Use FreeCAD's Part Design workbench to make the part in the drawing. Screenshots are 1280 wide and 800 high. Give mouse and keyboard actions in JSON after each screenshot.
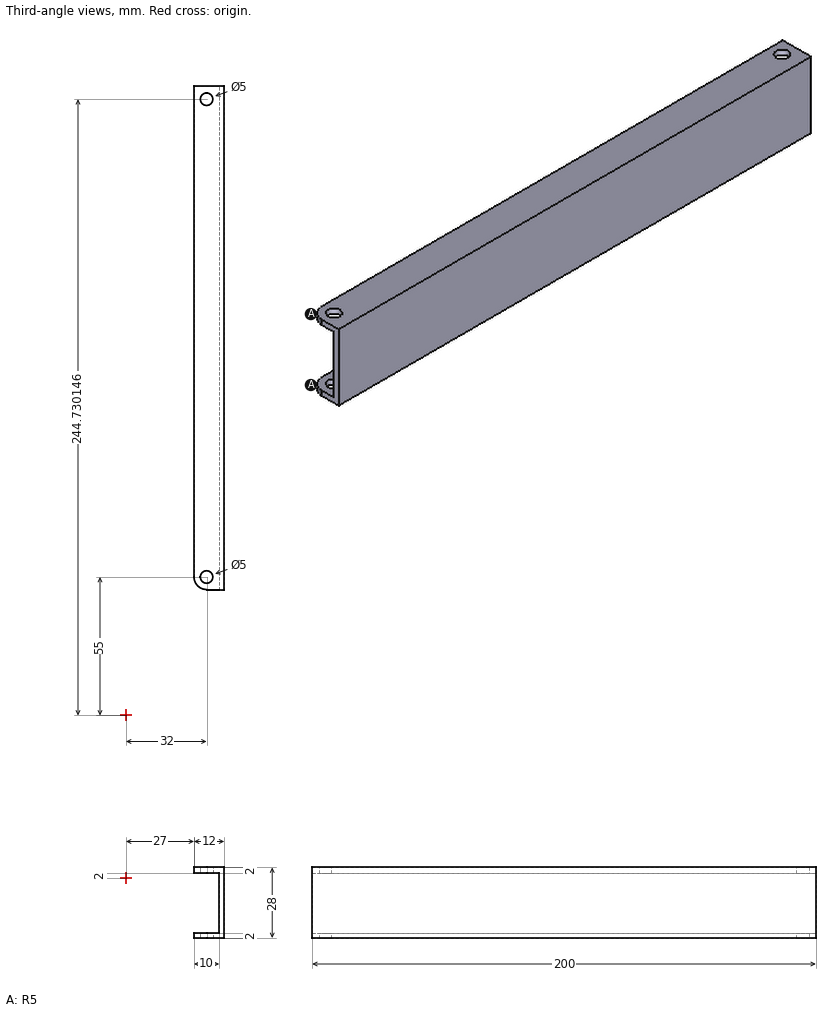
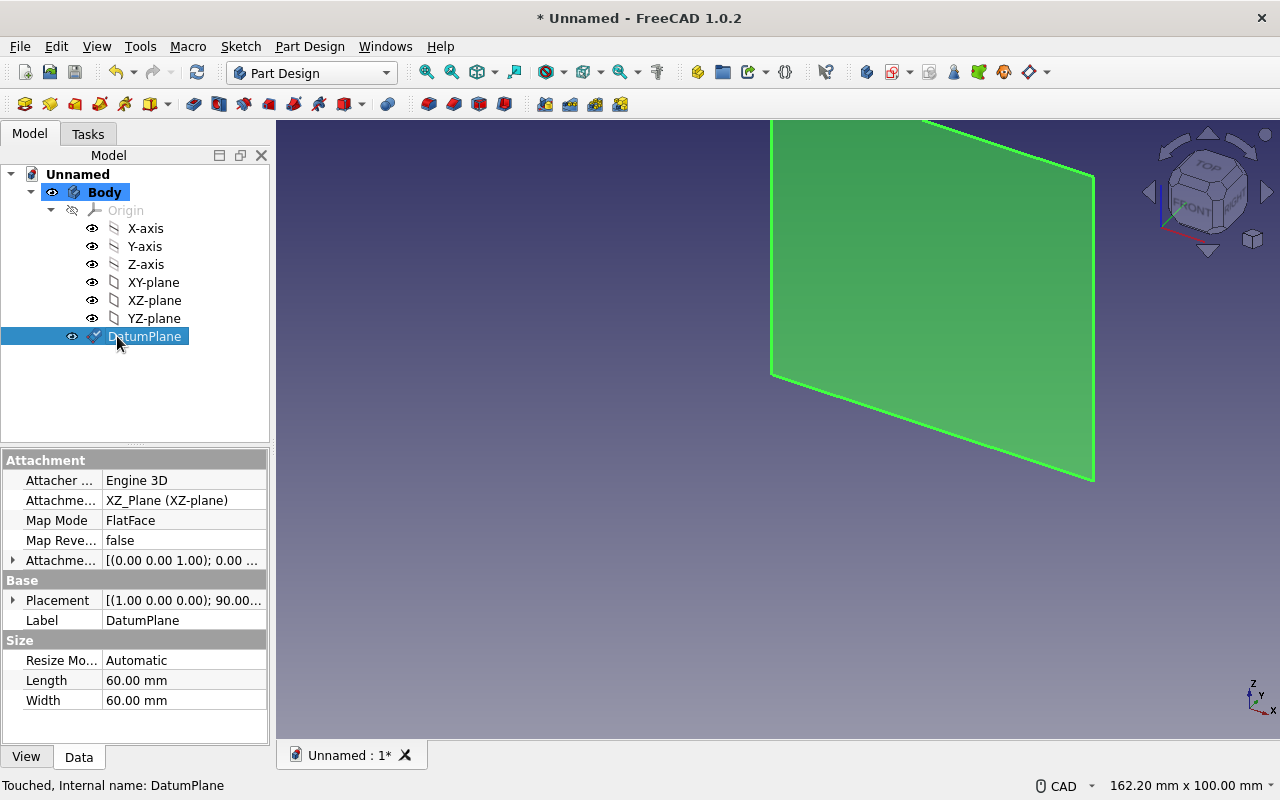
{"action": "left_click", "coordinate": [892, 72]}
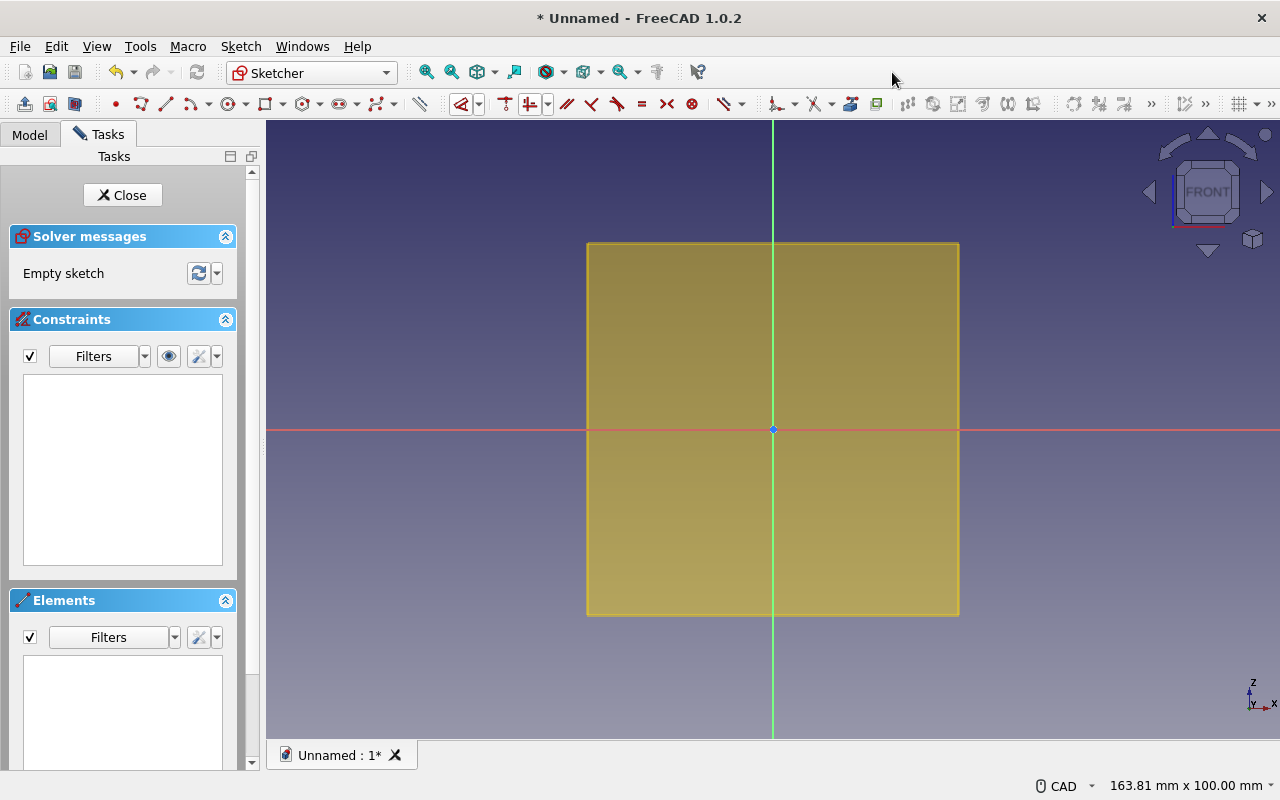
{"action": "scroll", "coordinate": [1048, 542], "scroll_direction": "up", "scroll_amount": 4}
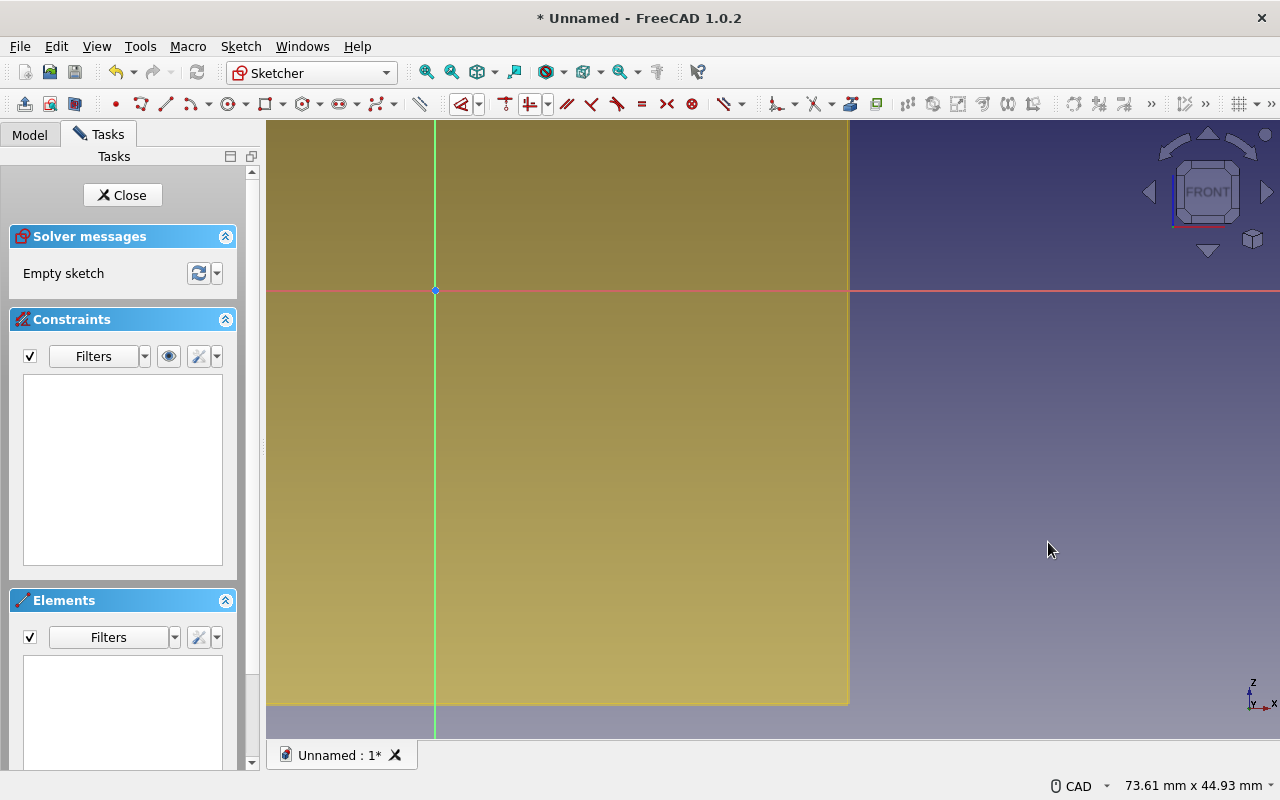
{"action": "left_click", "coordinate": [141, 104]}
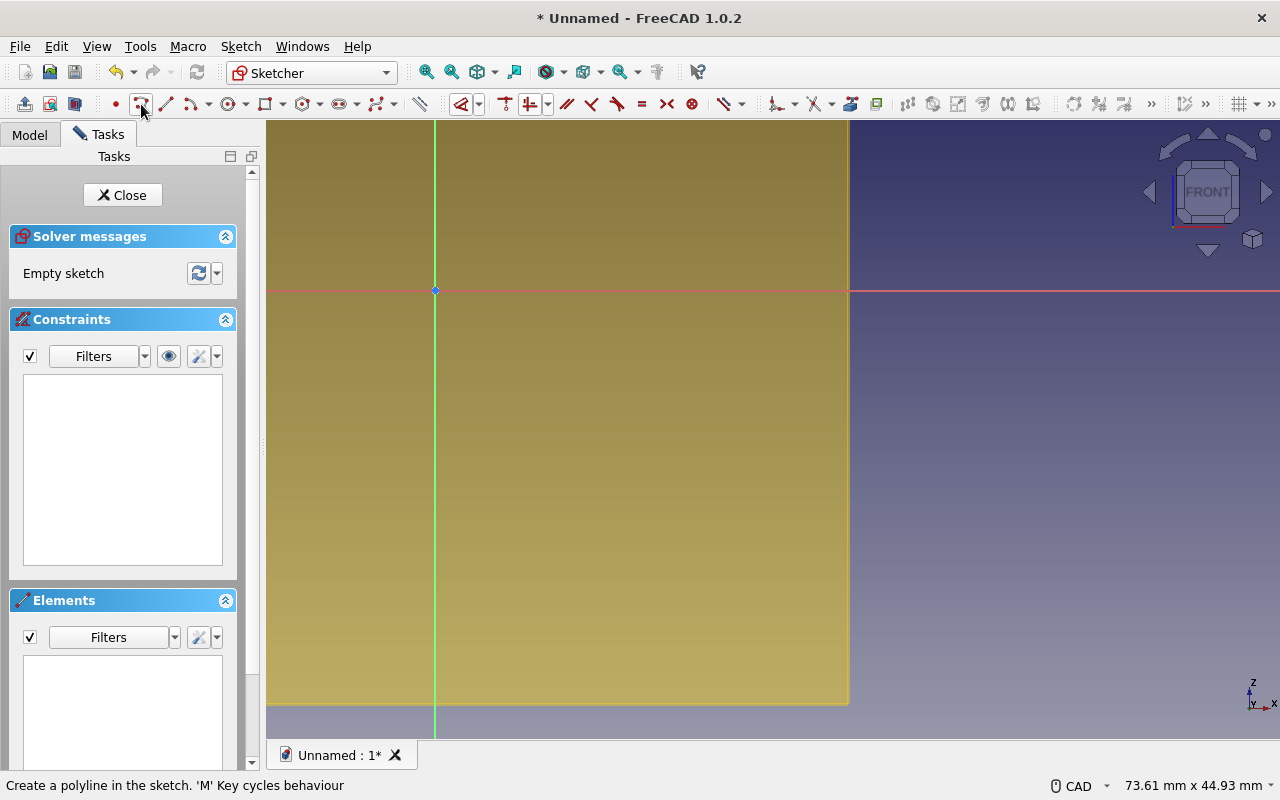
{"action": "left_click", "coordinate": [807, 263]}
{"action": "left_click", "coordinate": [807, 236]}
{"action": "left_click", "coordinate": [972, 236]}
{"action": "left_click", "coordinate": [972, 621]}
{"action": "left_click", "coordinate": [807, 621]}
{"action": "left_click", "coordinate": [807, 594]}
{"action": "left_click", "coordinate": [945, 594]}
{"action": "left_click", "coordinate": [945, 263]}
{"action": "left_click", "coordinate": [807, 264]}
{"action": "key", "text": "Escape"}
{"action": "key", "text": "Escape"}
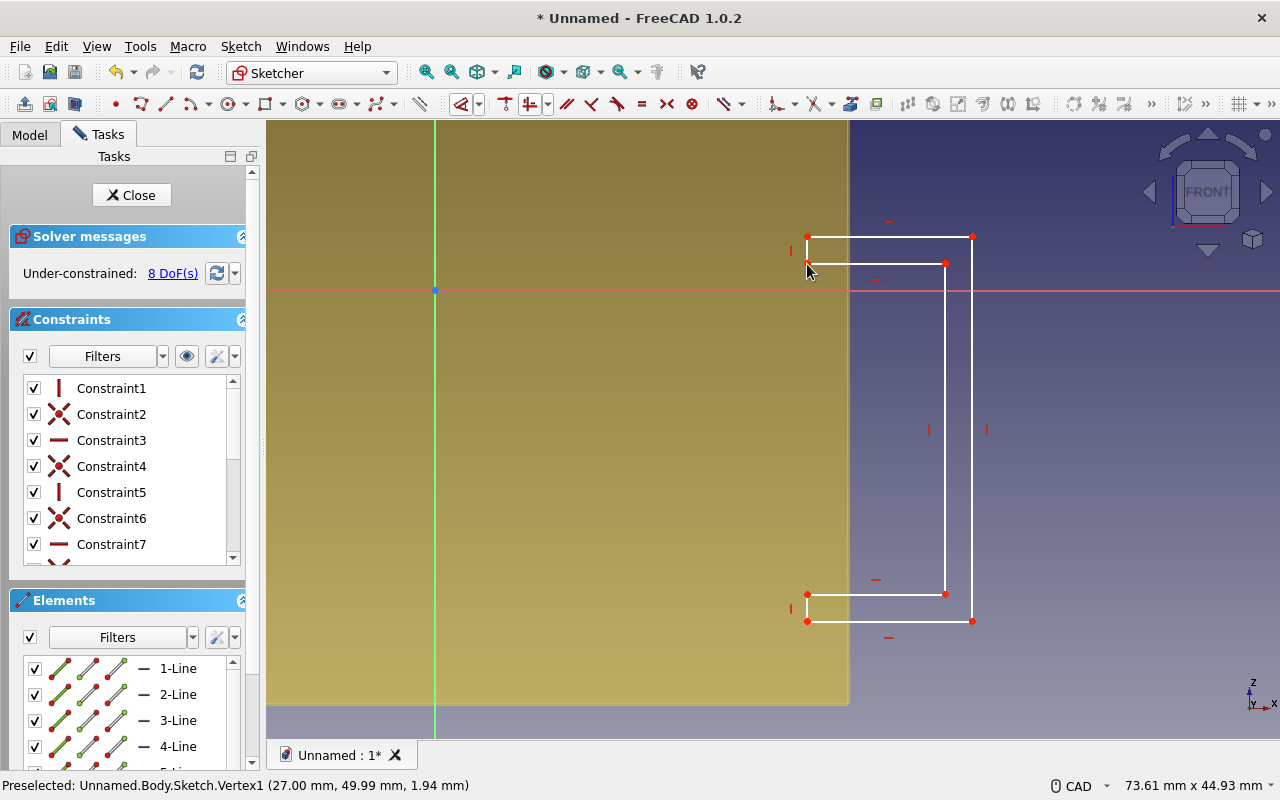
{"action": "scroll", "coordinate": [807, 253], "scroll_direction": "up", "scroll_amount": 2}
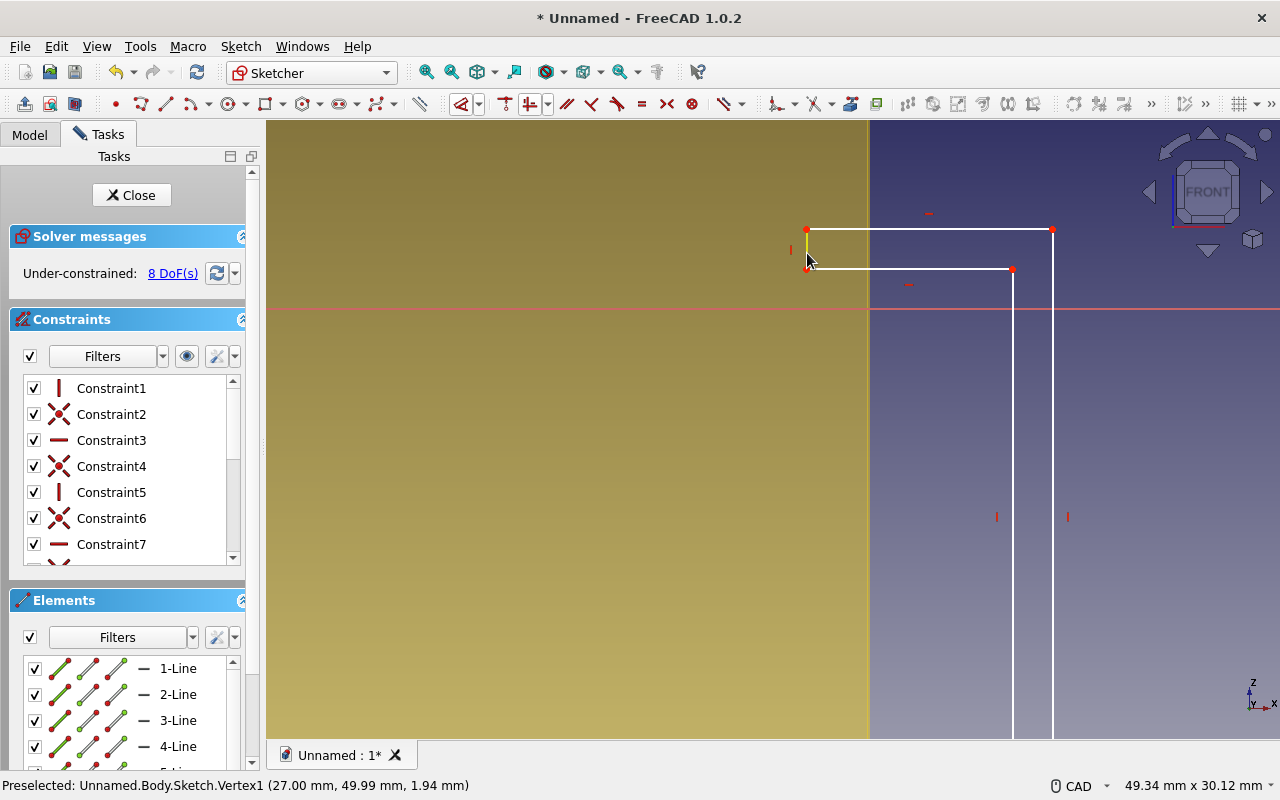
{"action": "left_click", "coordinate": [807, 253]}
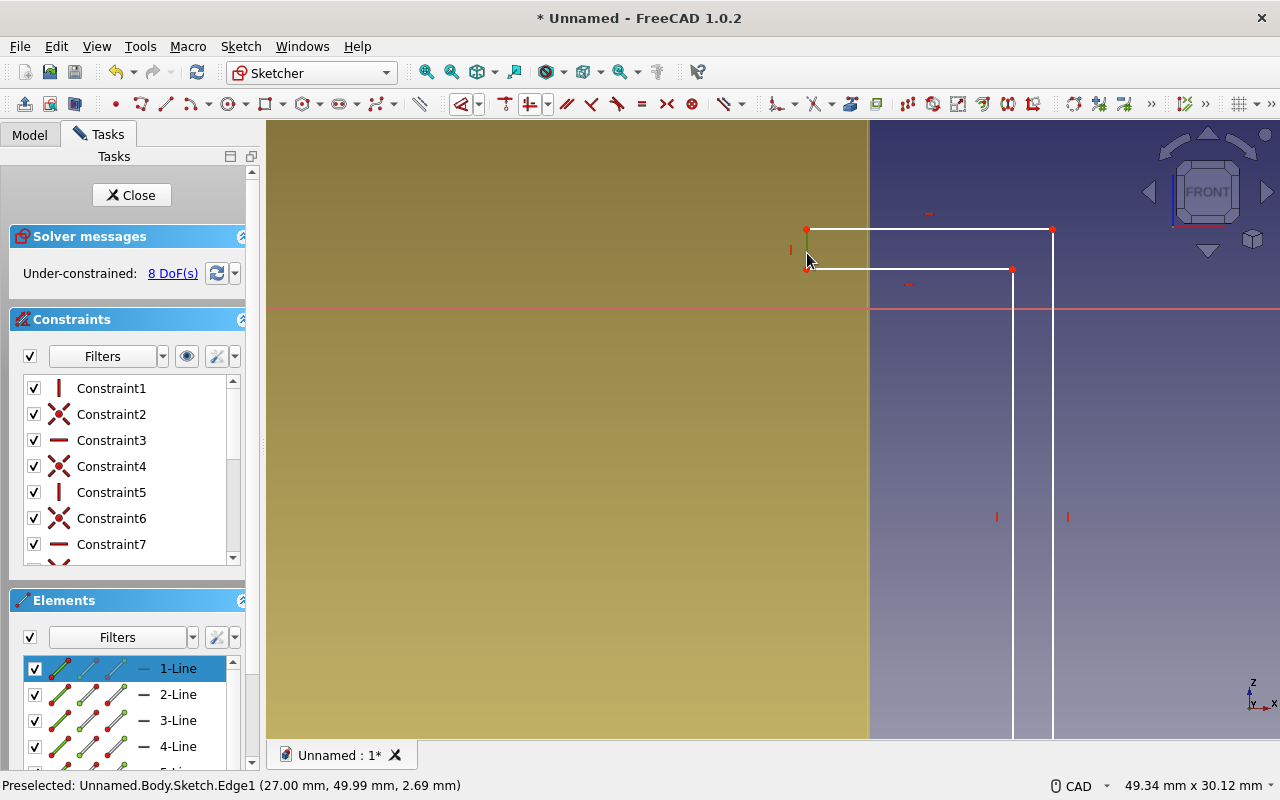
{"action": "left_click", "coordinate": [478, 104]}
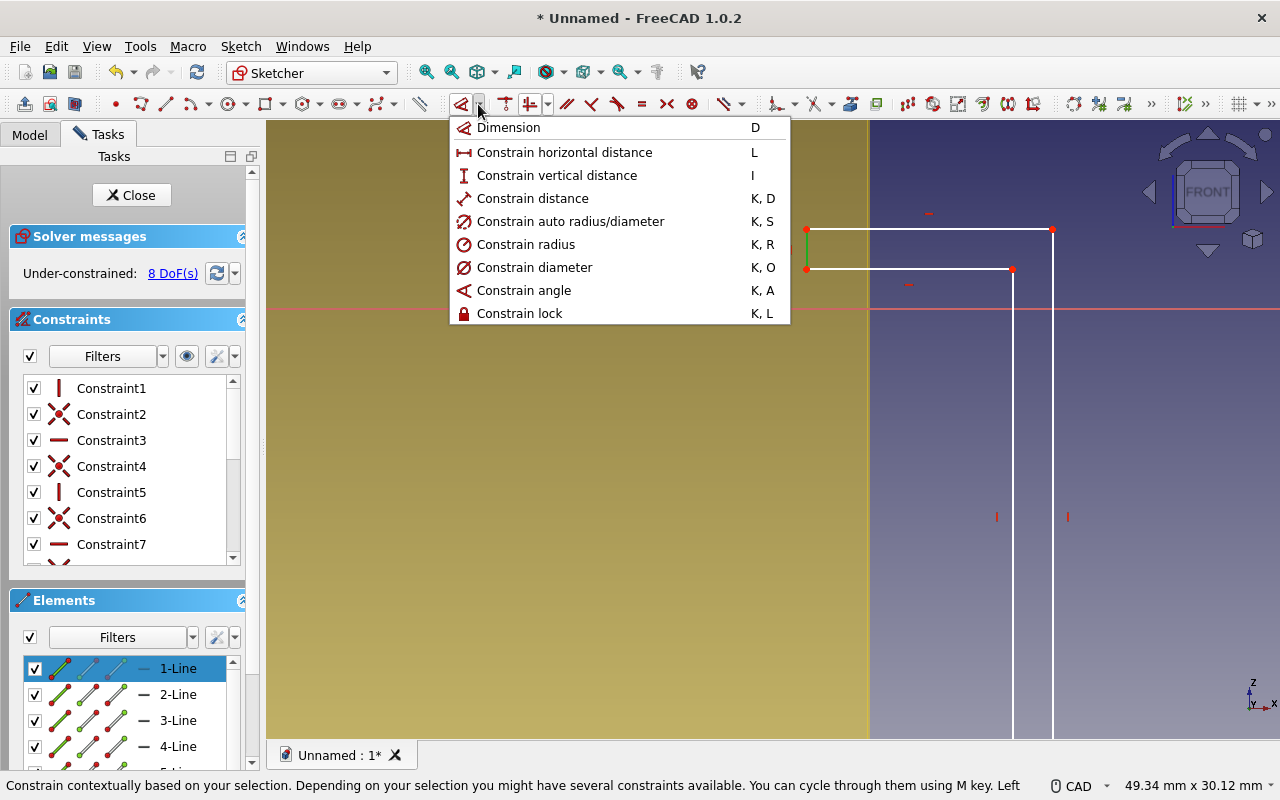
{"action": "left_click", "coordinate": [620, 176]}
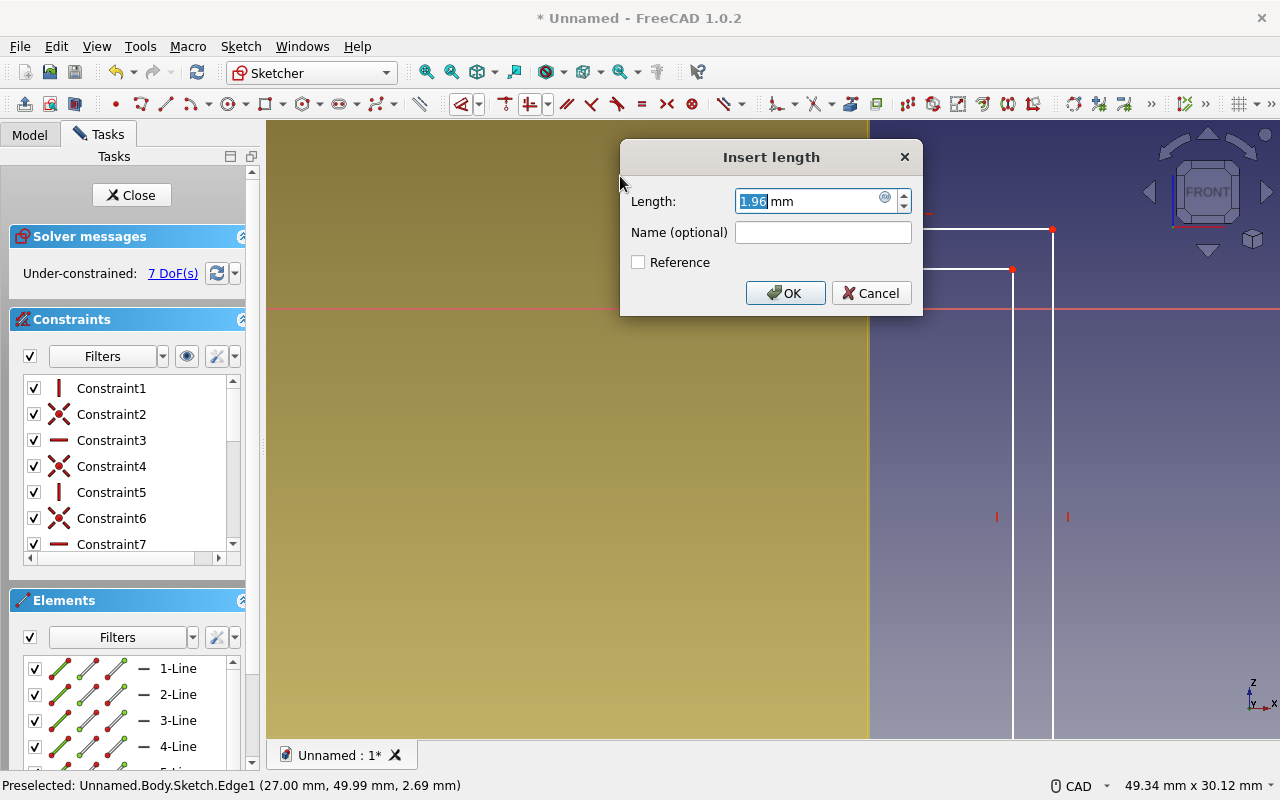
{"action": "type", "text": "2"}
{"action": "key", "text": "Return"}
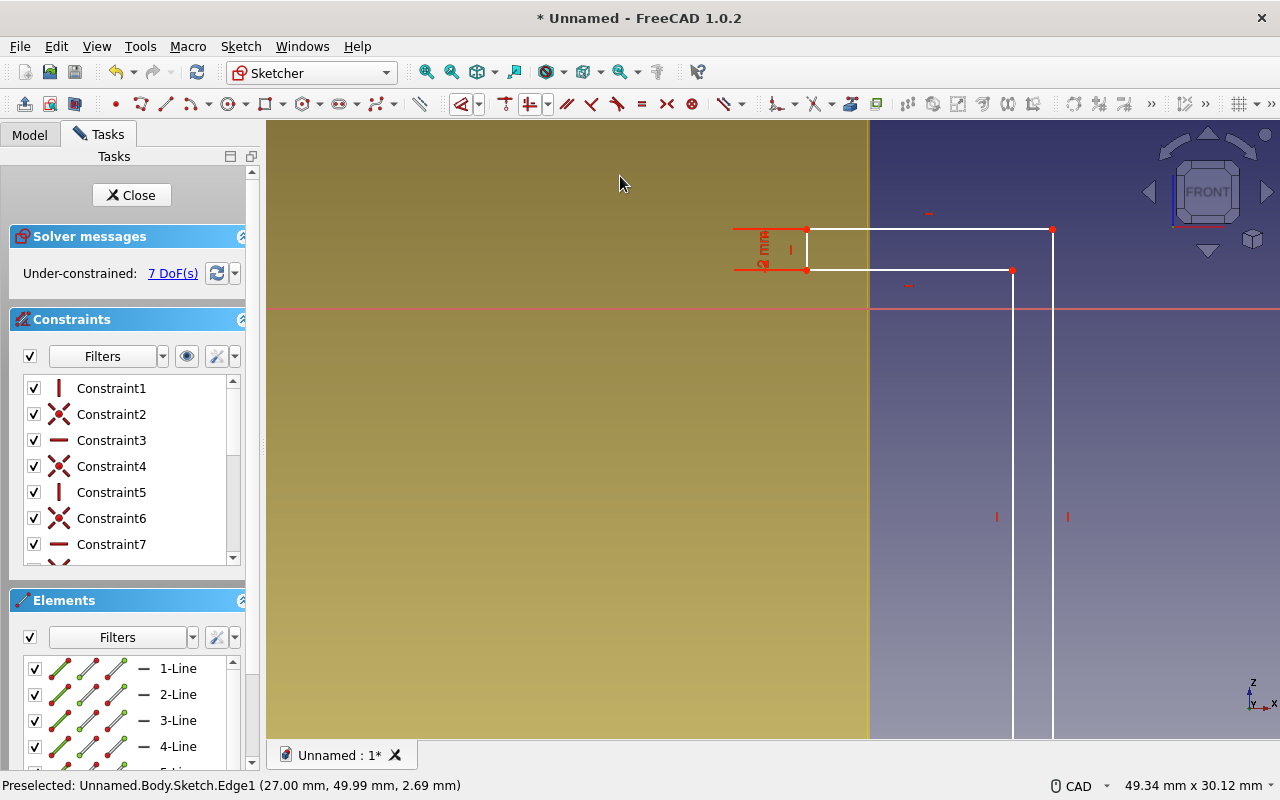
{"action": "scroll", "coordinate": [810, 256], "scroll_direction": "down", "scroll_amount": 2}